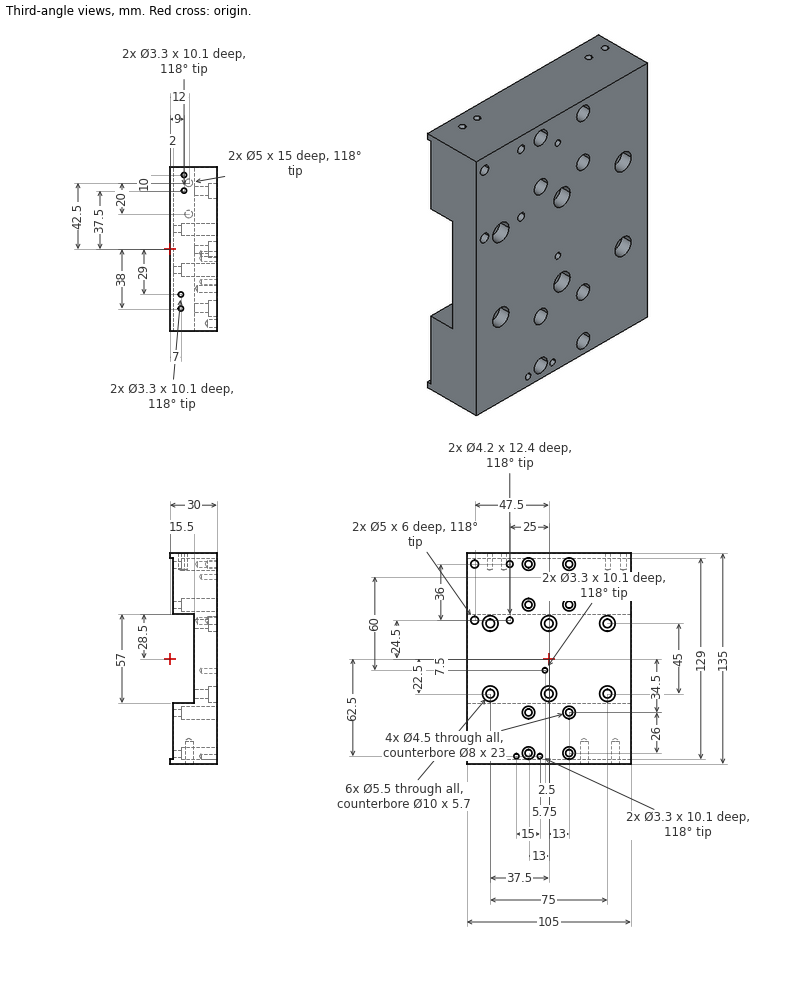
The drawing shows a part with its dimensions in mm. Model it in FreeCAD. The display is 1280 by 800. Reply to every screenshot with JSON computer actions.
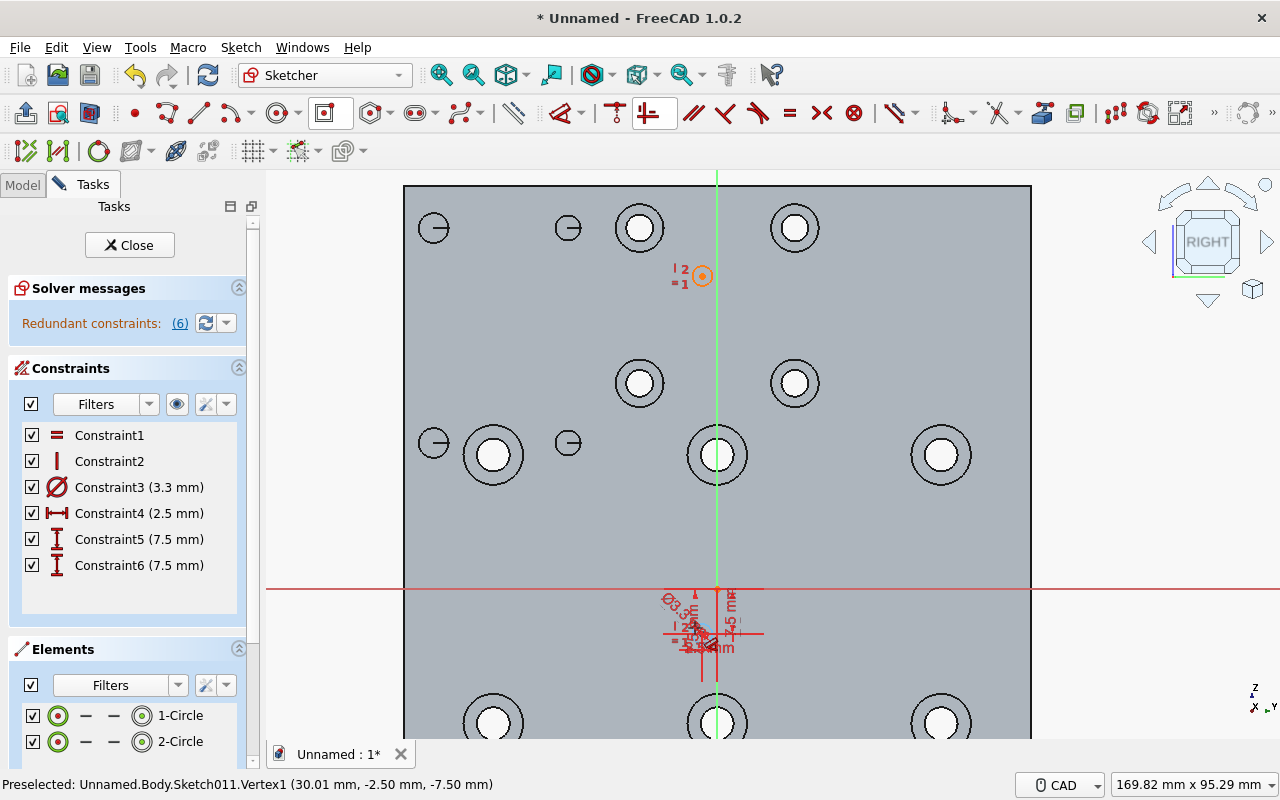
{"action": "left_click", "coordinate": [702, 276]}
{"action": "left_click", "coordinate": [668, 455]}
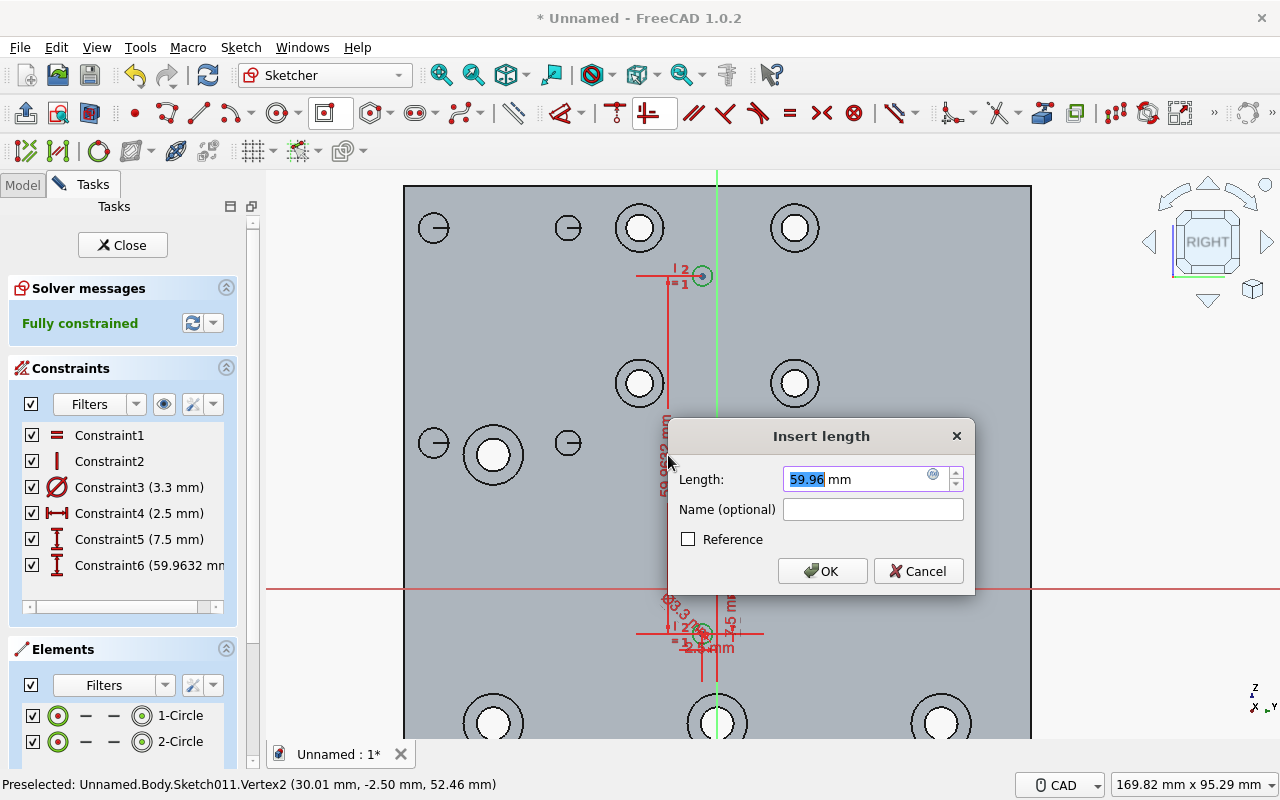
{"action": "type", "text": "60"}
{"action": "key", "text": "Return"}
{"action": "key", "text": "Escape"}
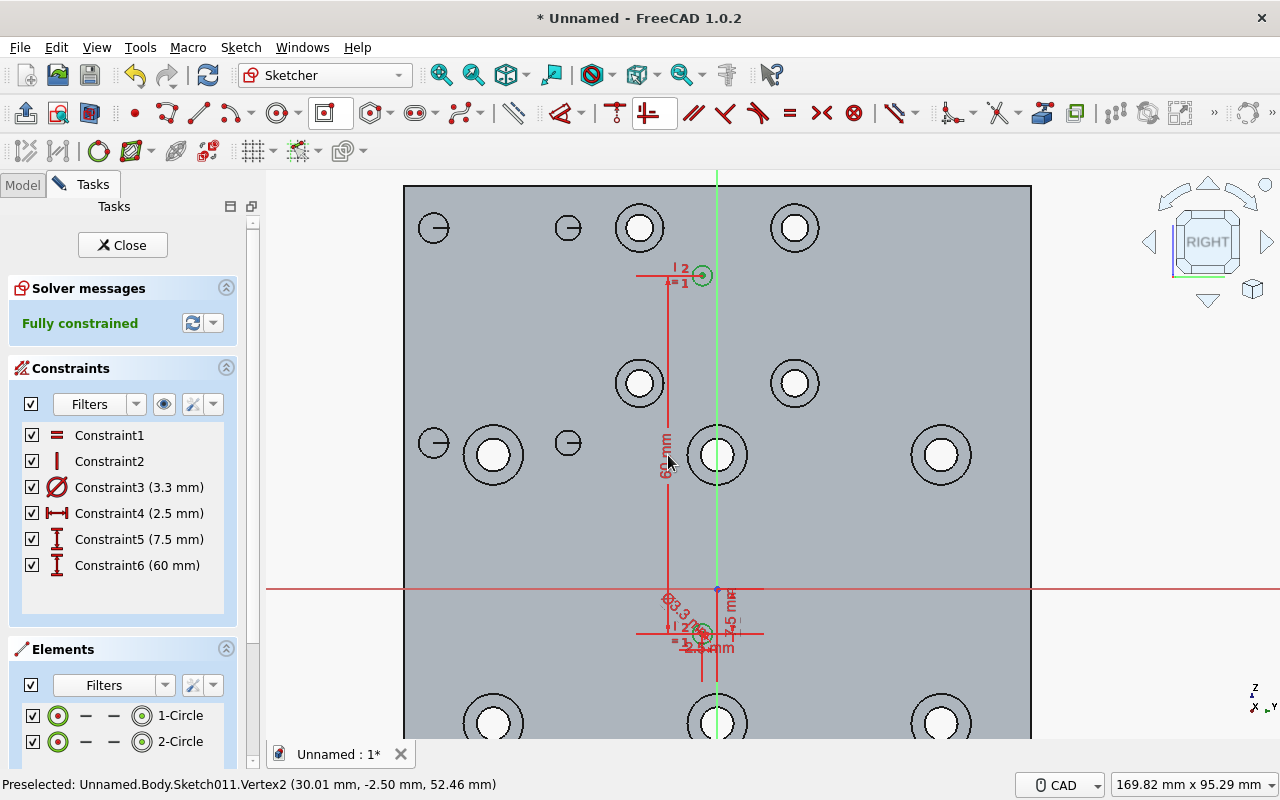
{"action": "left_click", "coordinate": [123, 245]}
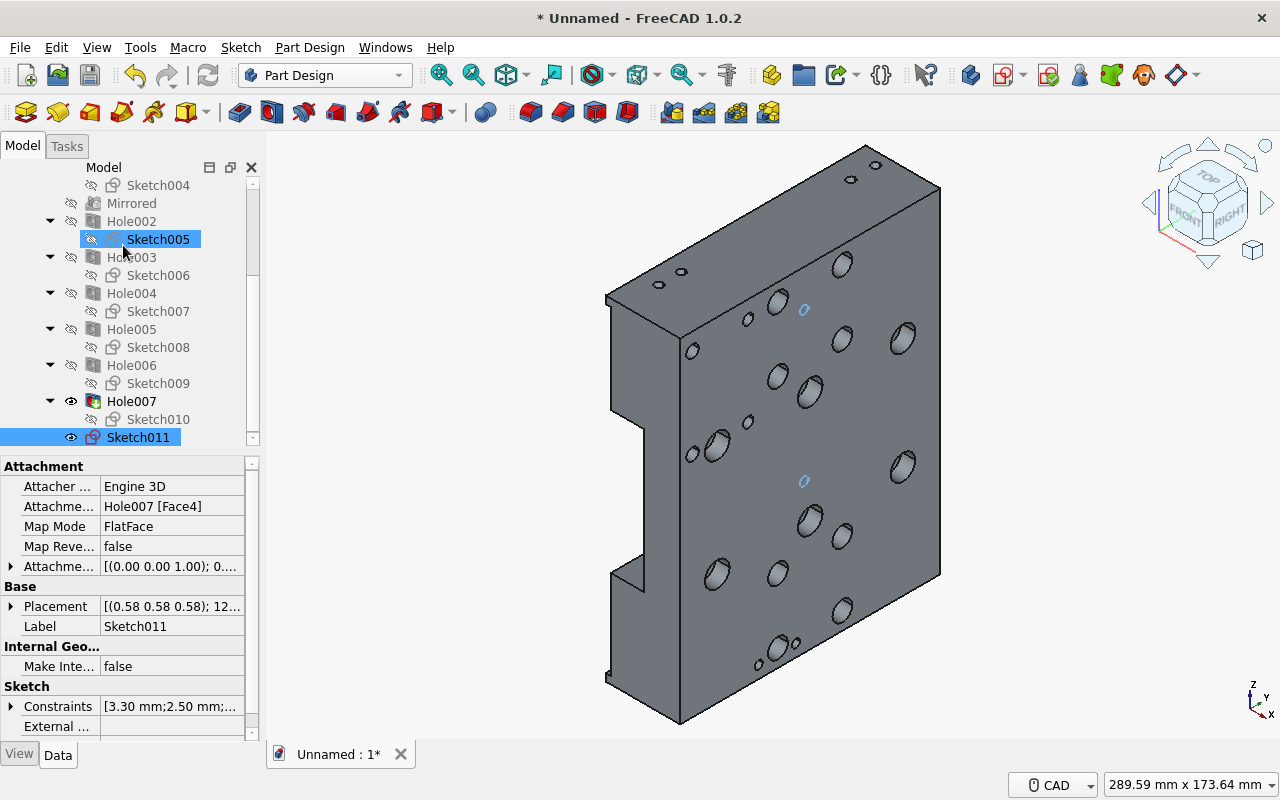
{"action": "left_click", "coordinate": [272, 112]}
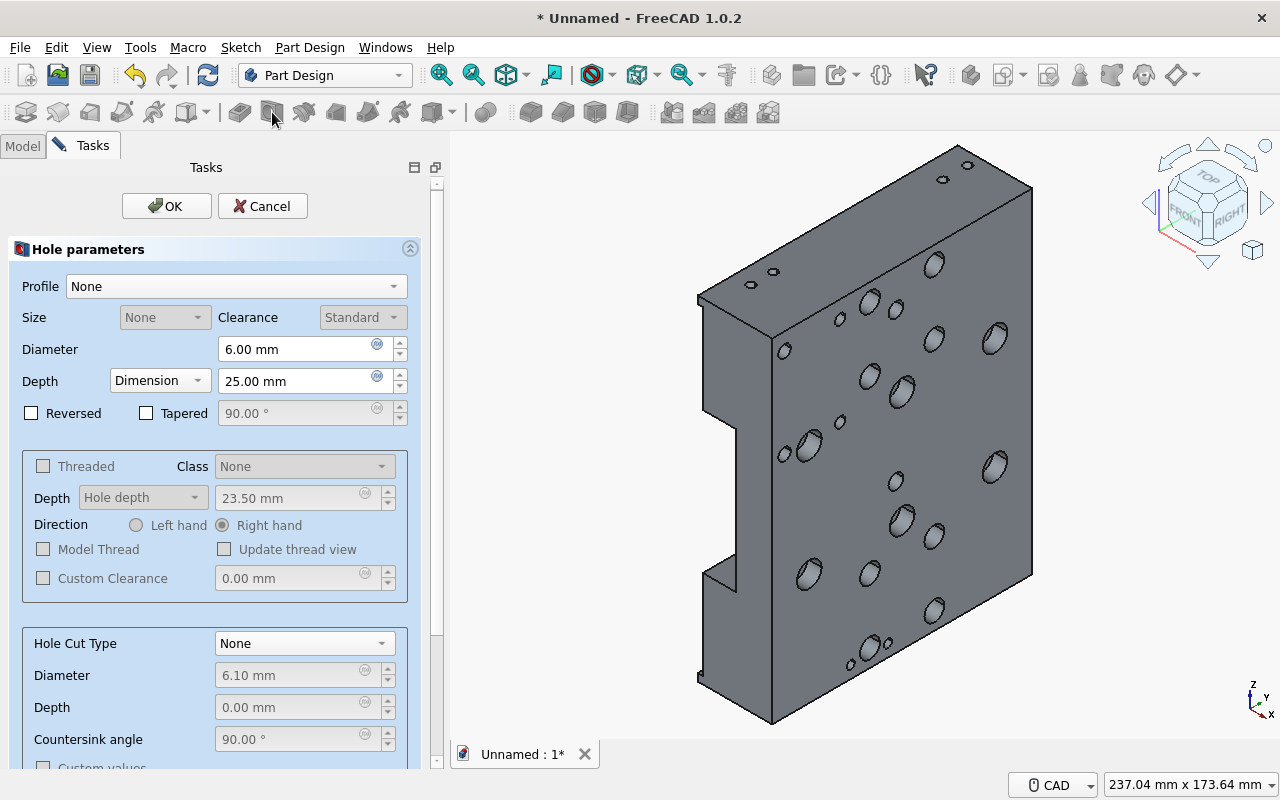
{"action": "triple_click", "coordinate": [305, 349]}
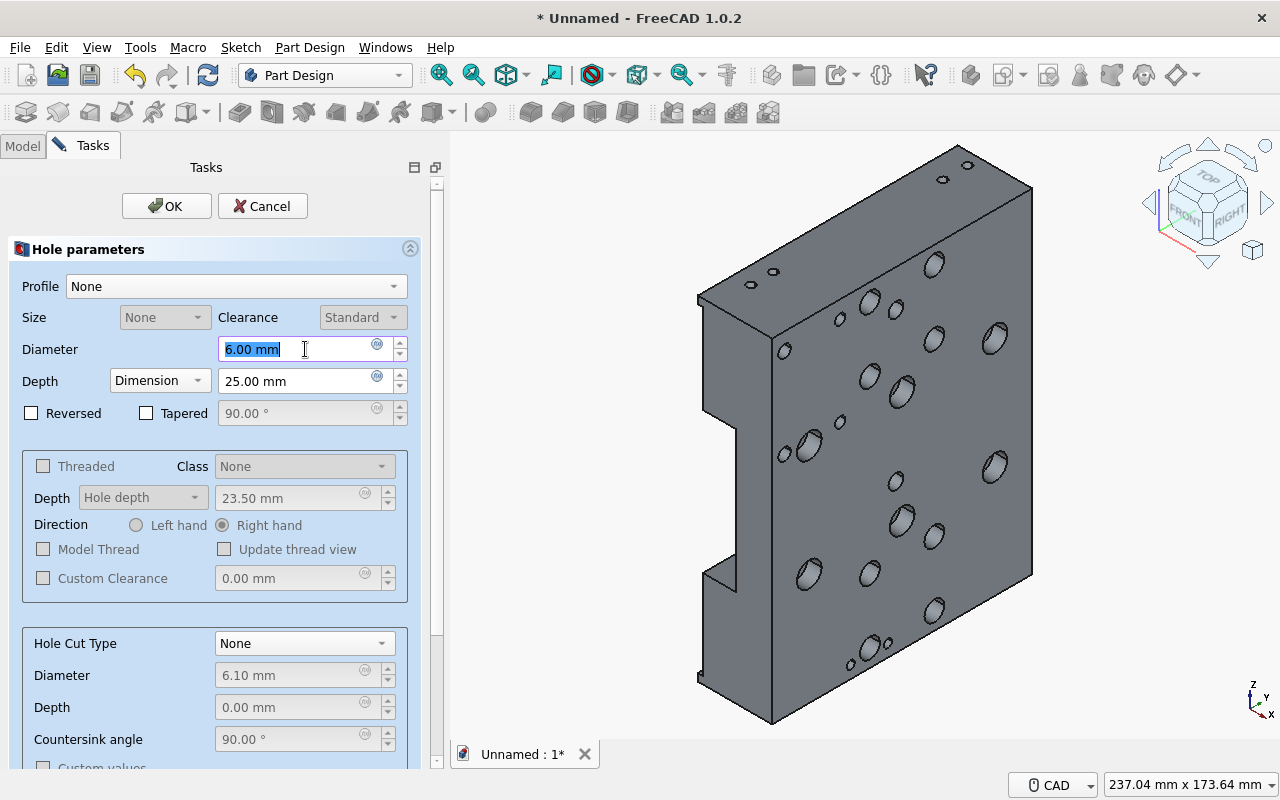
{"action": "type", "text": "3.3"}
{"action": "key", "text": "Tab"}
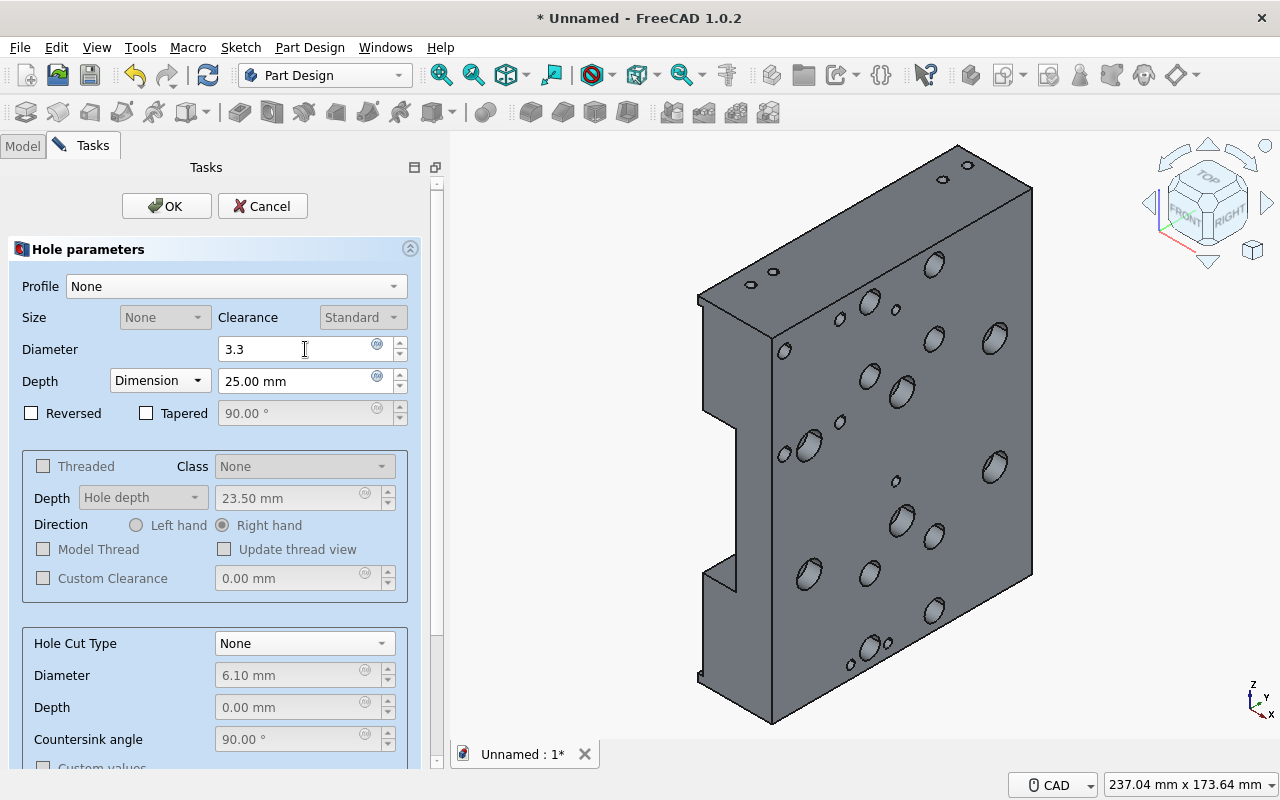
{"action": "triple_click", "coordinate": [305, 381]}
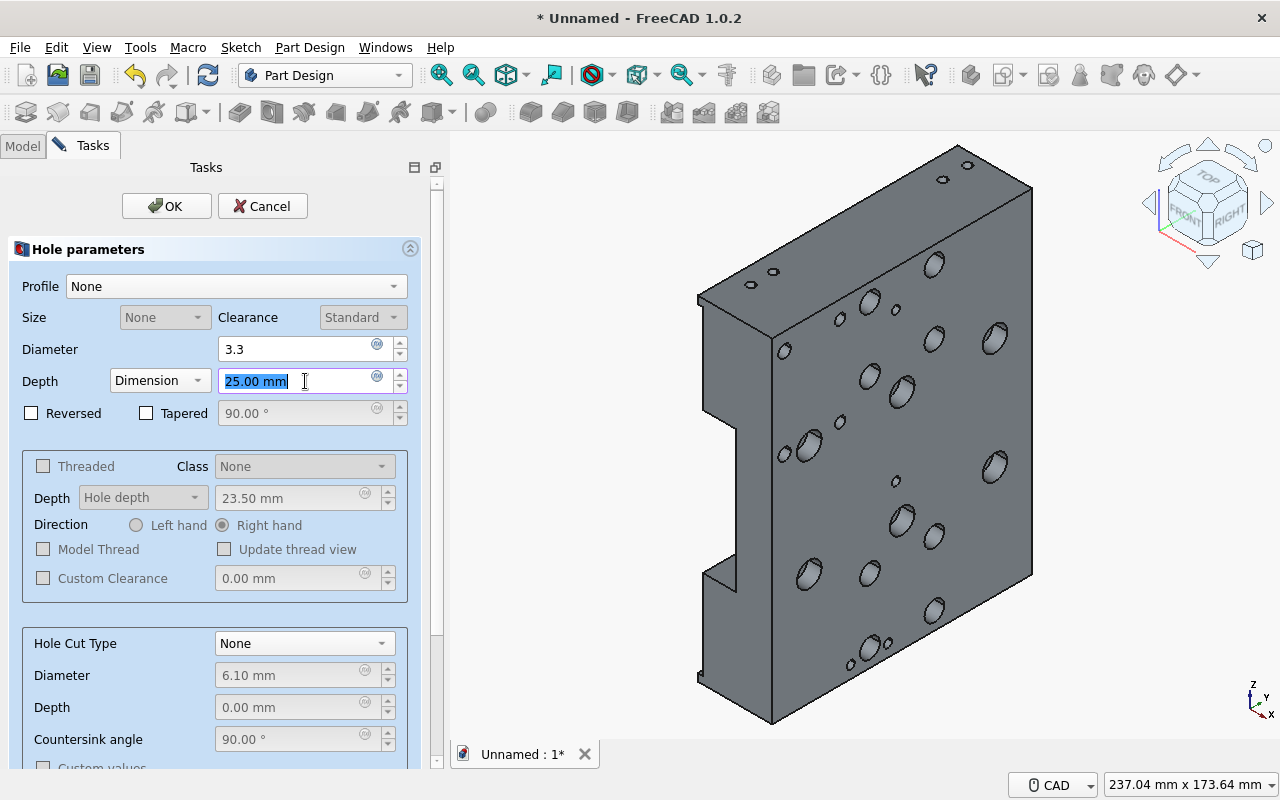
{"action": "type", "text": "10.1"}
{"action": "key", "text": "Tab"}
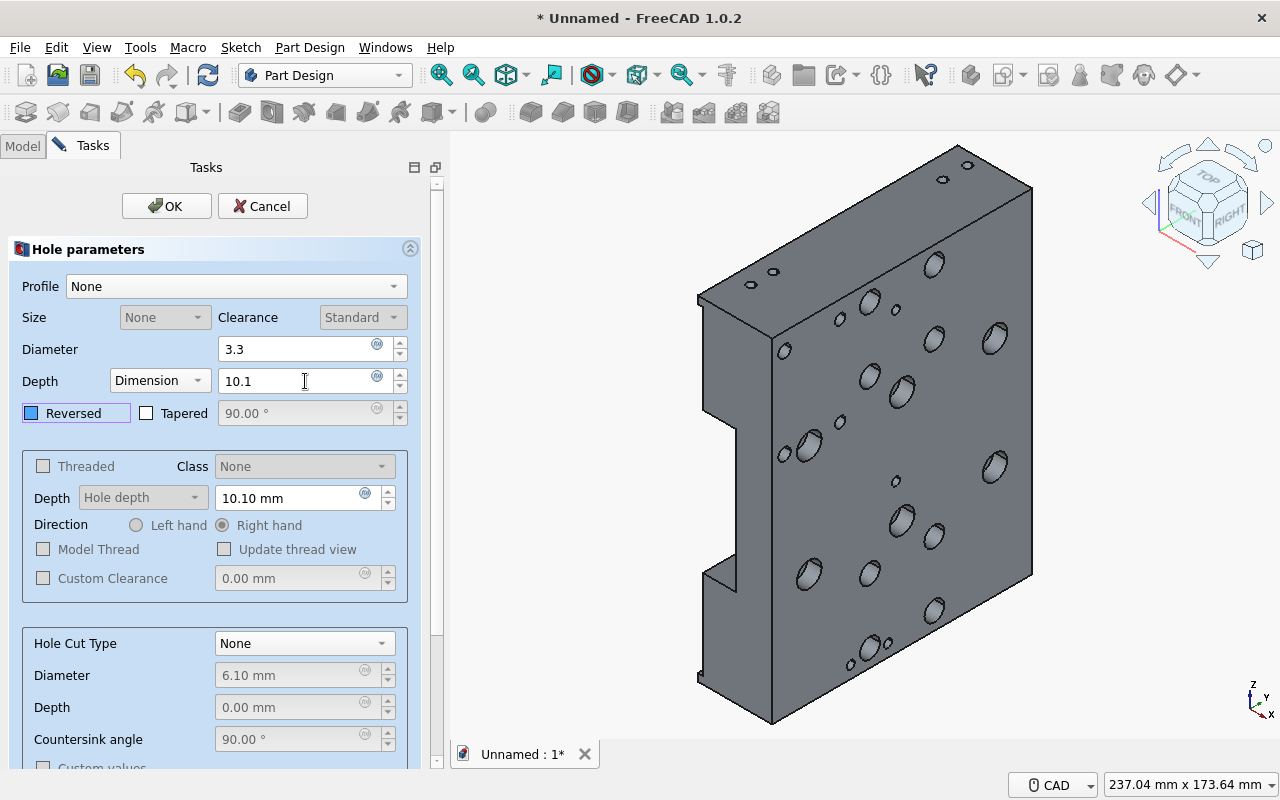
{"action": "left_click", "coordinate": [167, 206]}